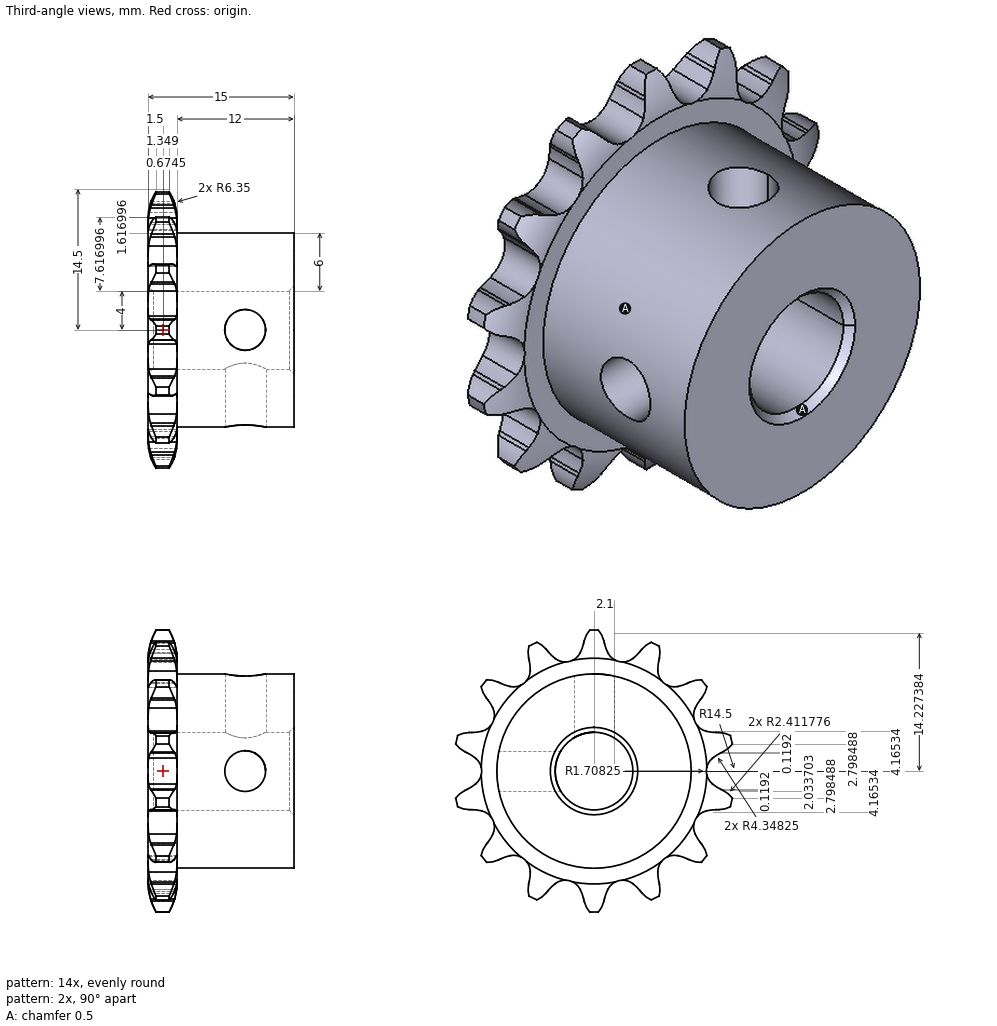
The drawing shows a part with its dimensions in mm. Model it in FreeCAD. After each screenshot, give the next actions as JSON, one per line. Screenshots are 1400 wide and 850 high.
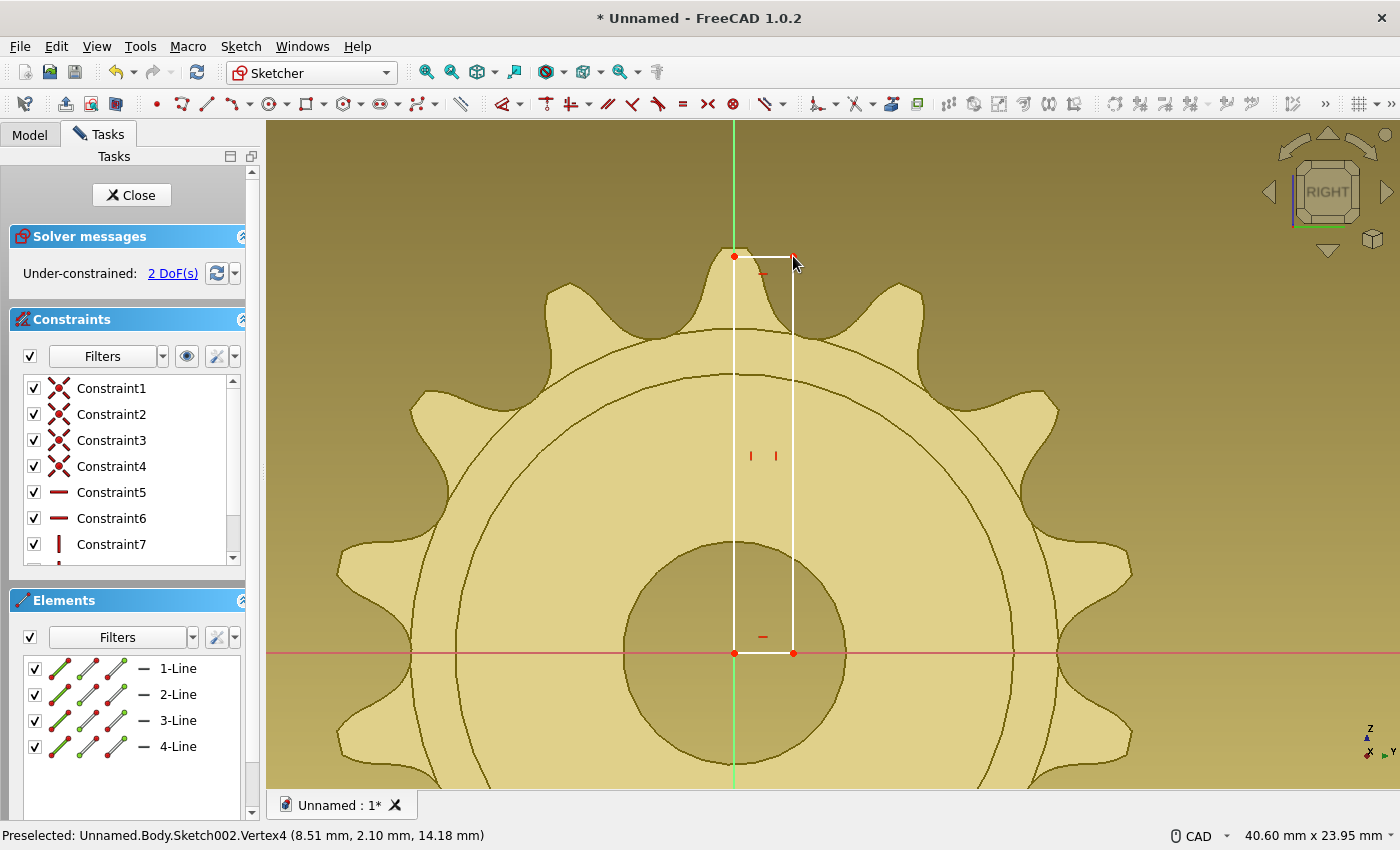
{"action": "left_click", "coordinate": [502, 104]}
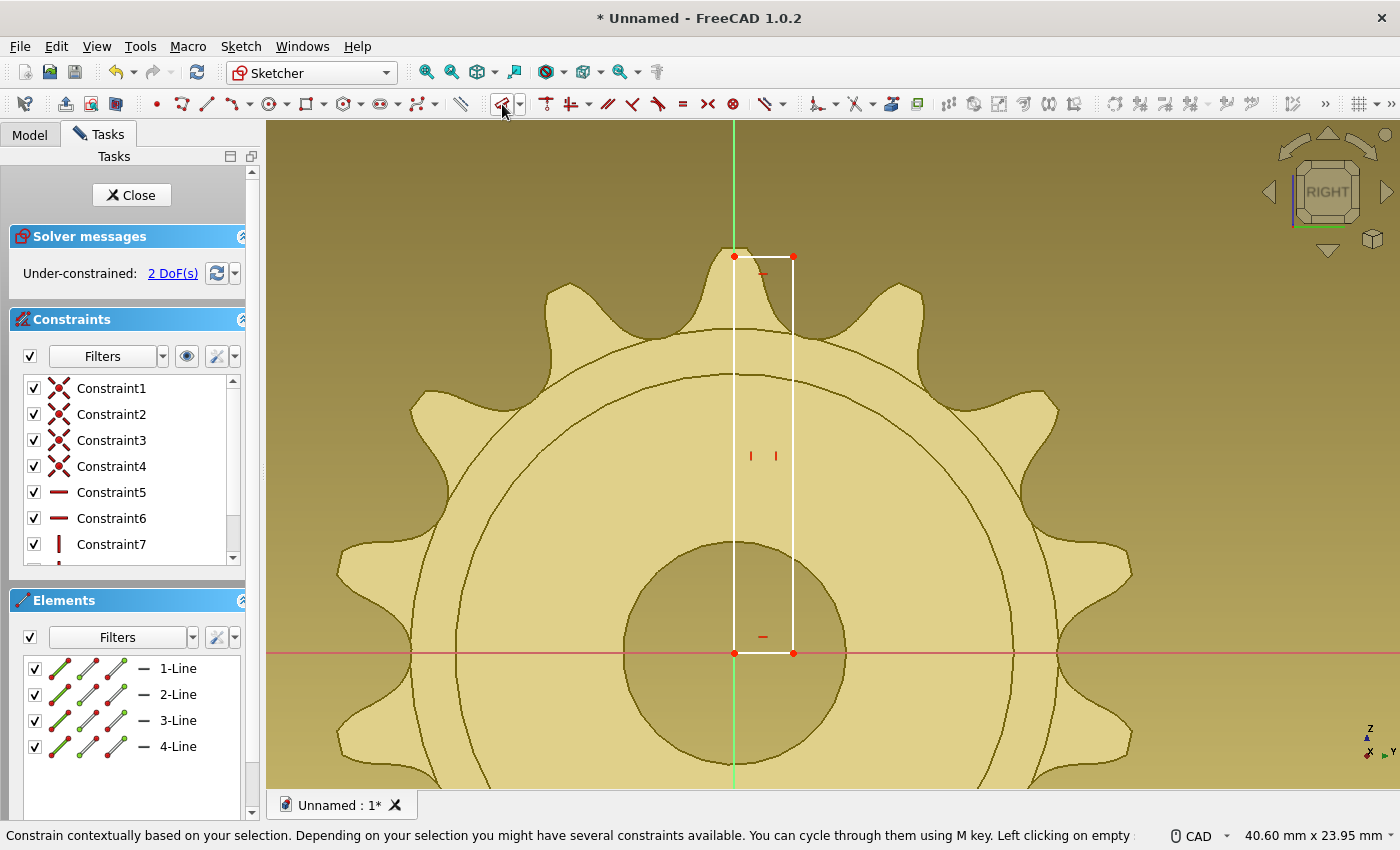
{"action": "left_click", "coordinate": [752, 653]}
{"action": "left_click", "coordinate": [764, 687]}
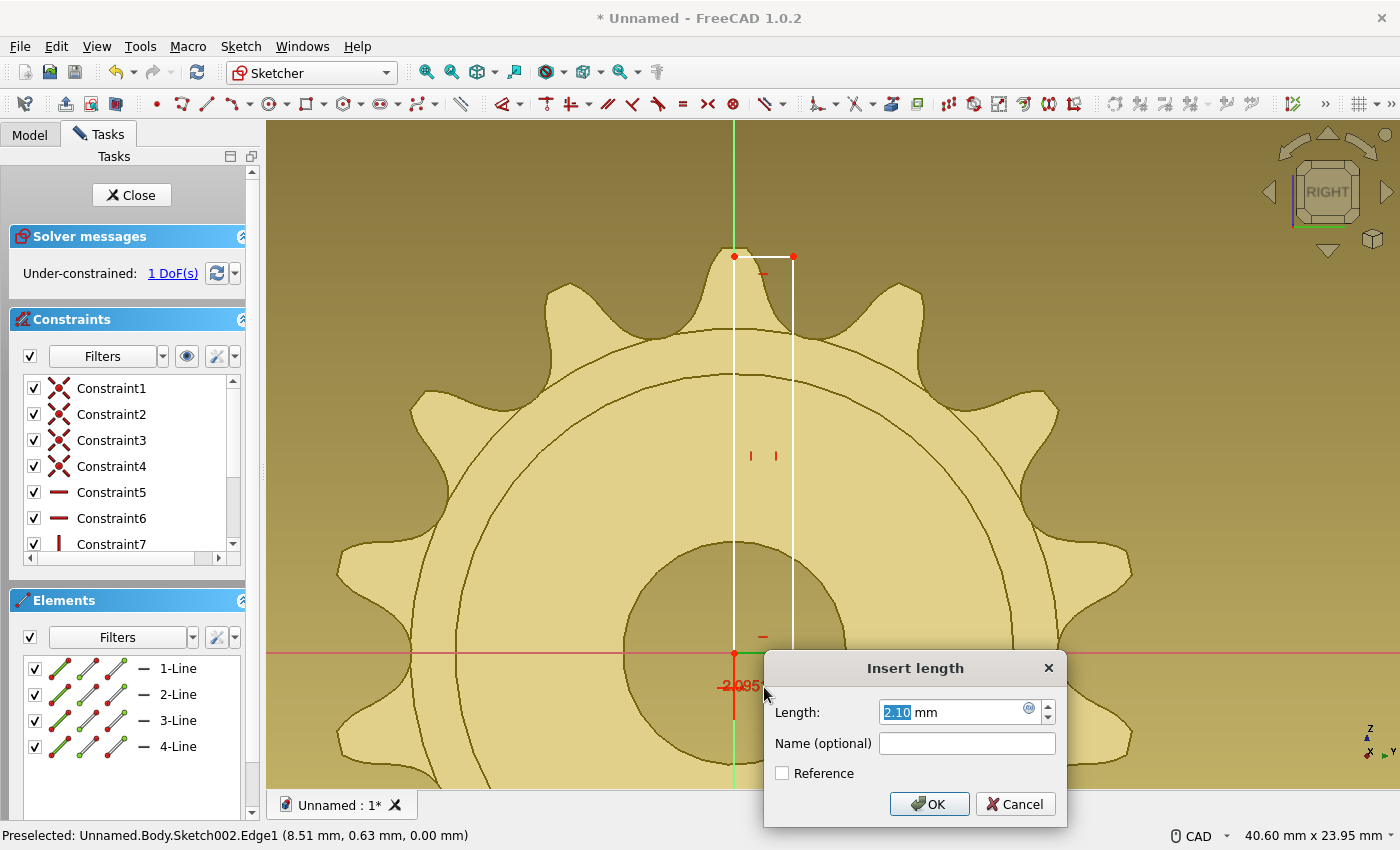
{"action": "type", "text": "2.1"}
{"action": "key", "text": "Return"}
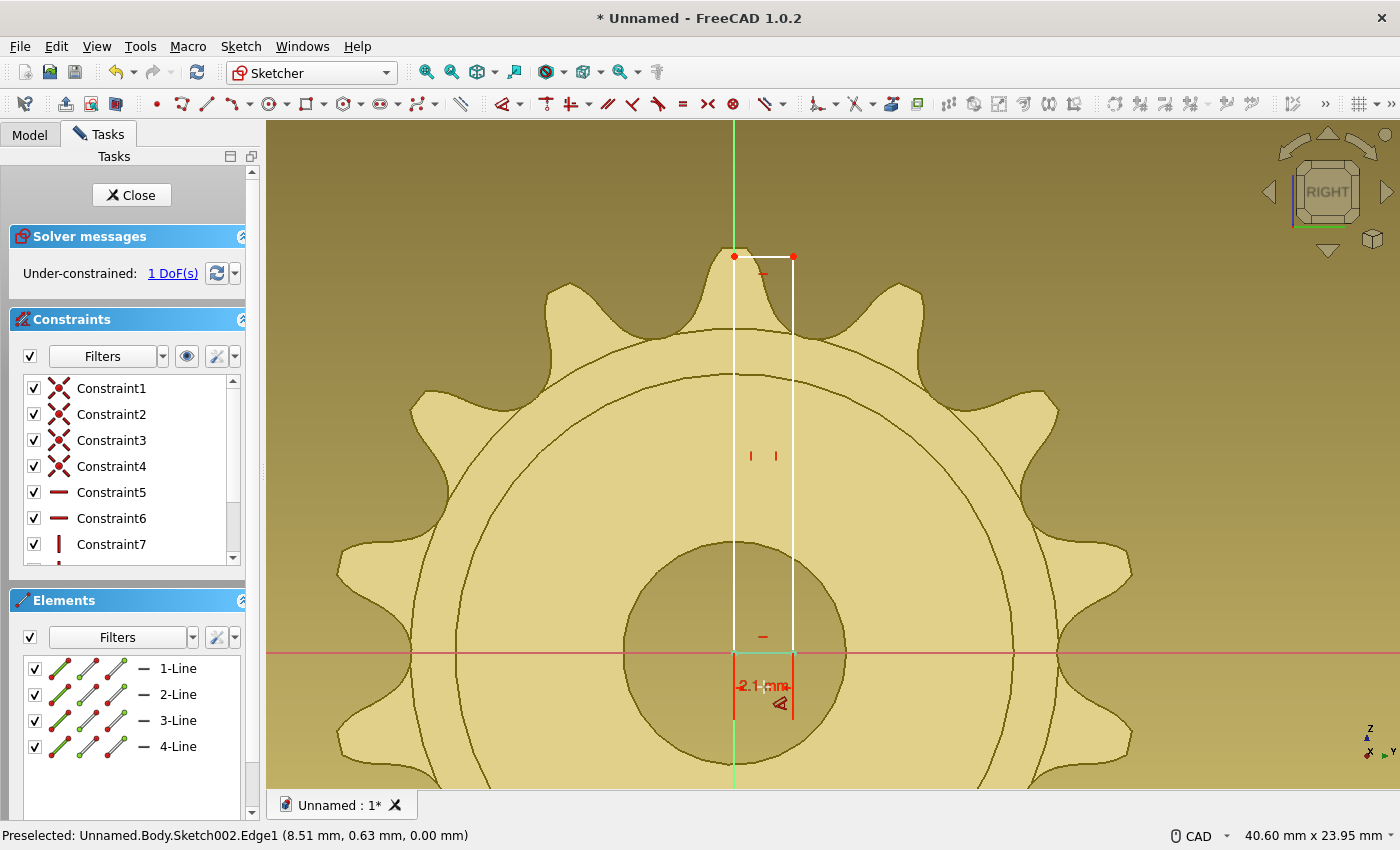
{"action": "left_click", "coordinate": [793, 534]}
{"action": "left_click", "coordinate": [827, 455]}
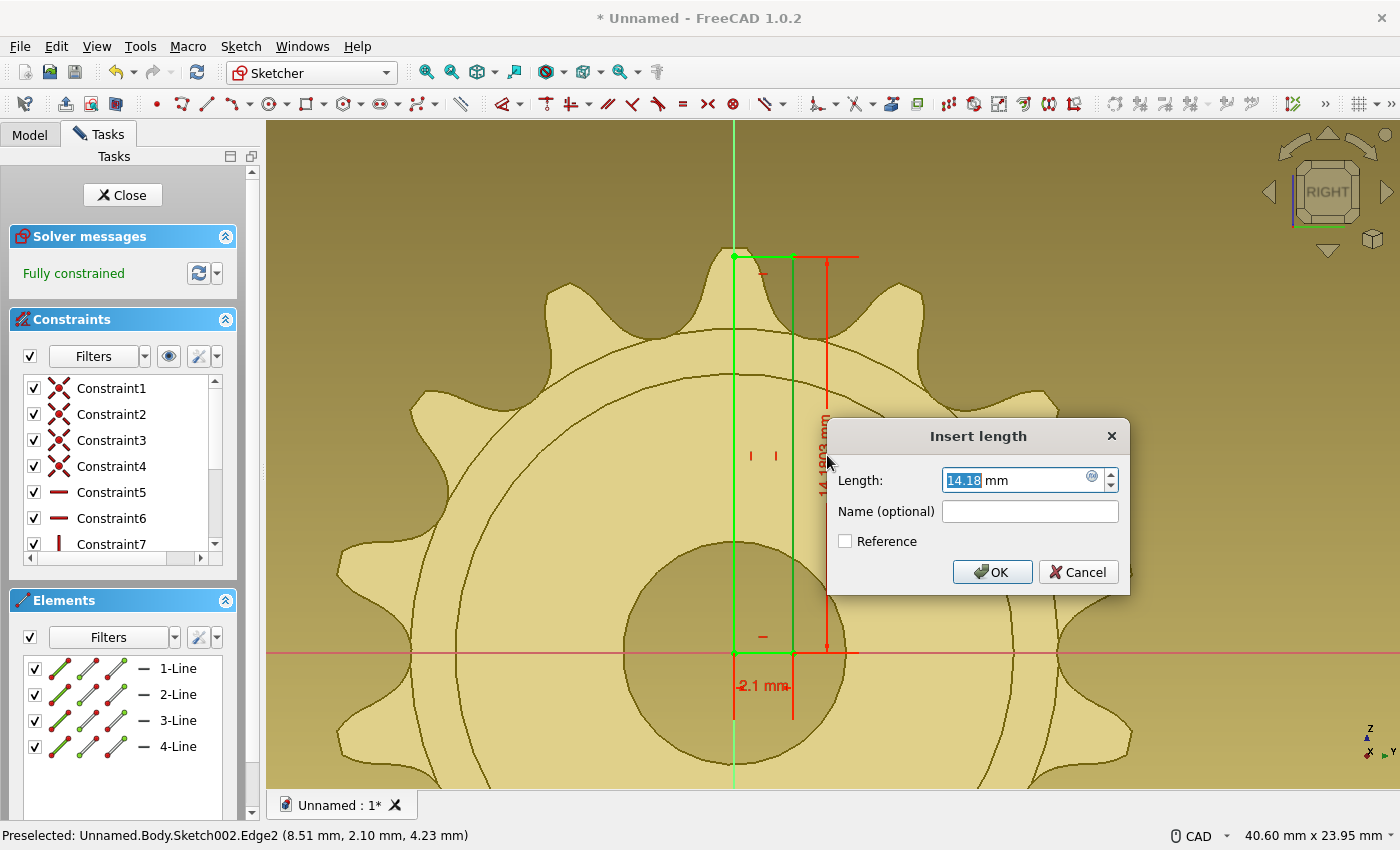
{"action": "type", "text": "14.227384"}
{"action": "key", "text": "Return"}
{"action": "key", "text": "Escape"}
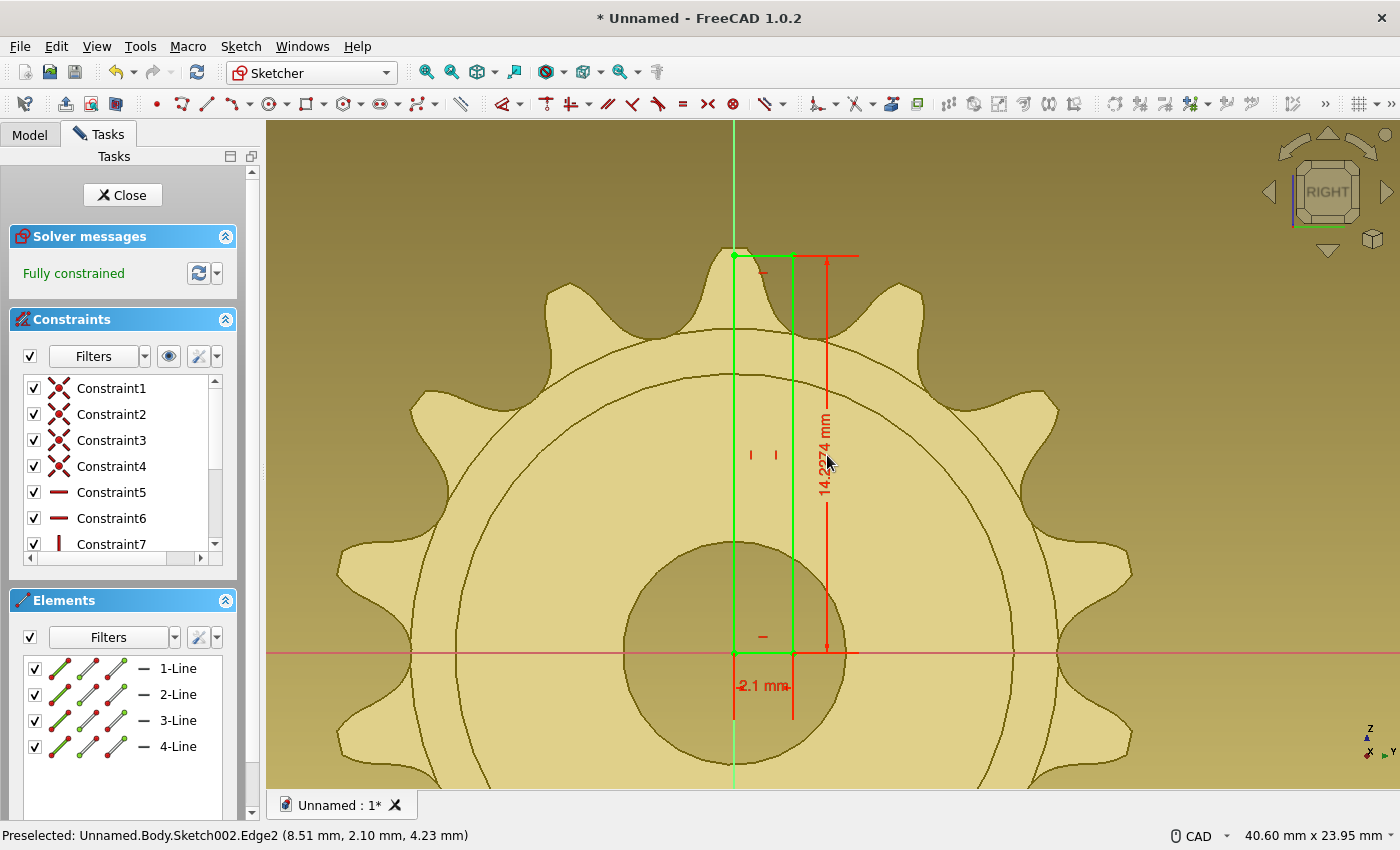
{"action": "left_click", "coordinate": [123, 195]}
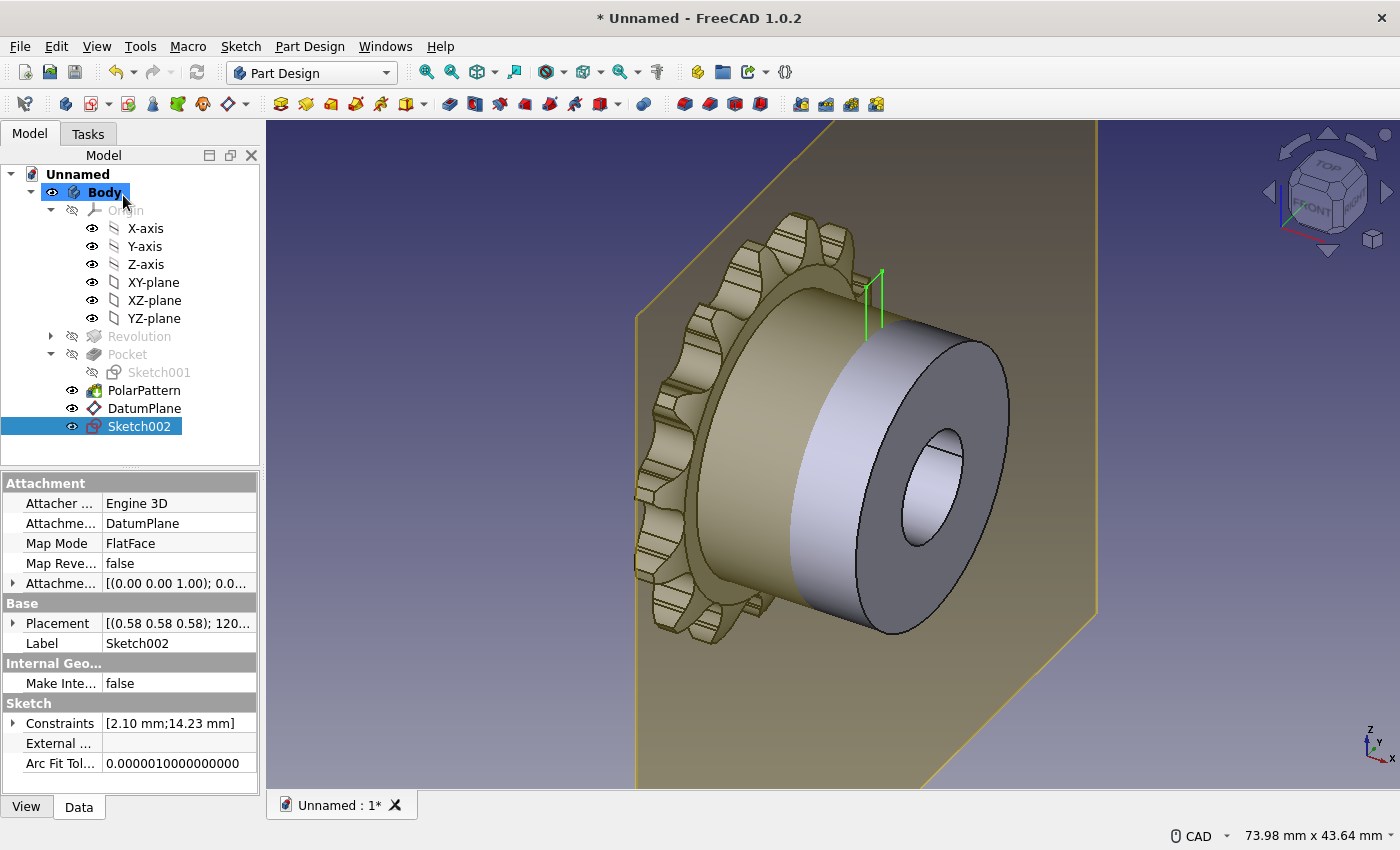
{"action": "left_click", "coordinate": [500, 104]}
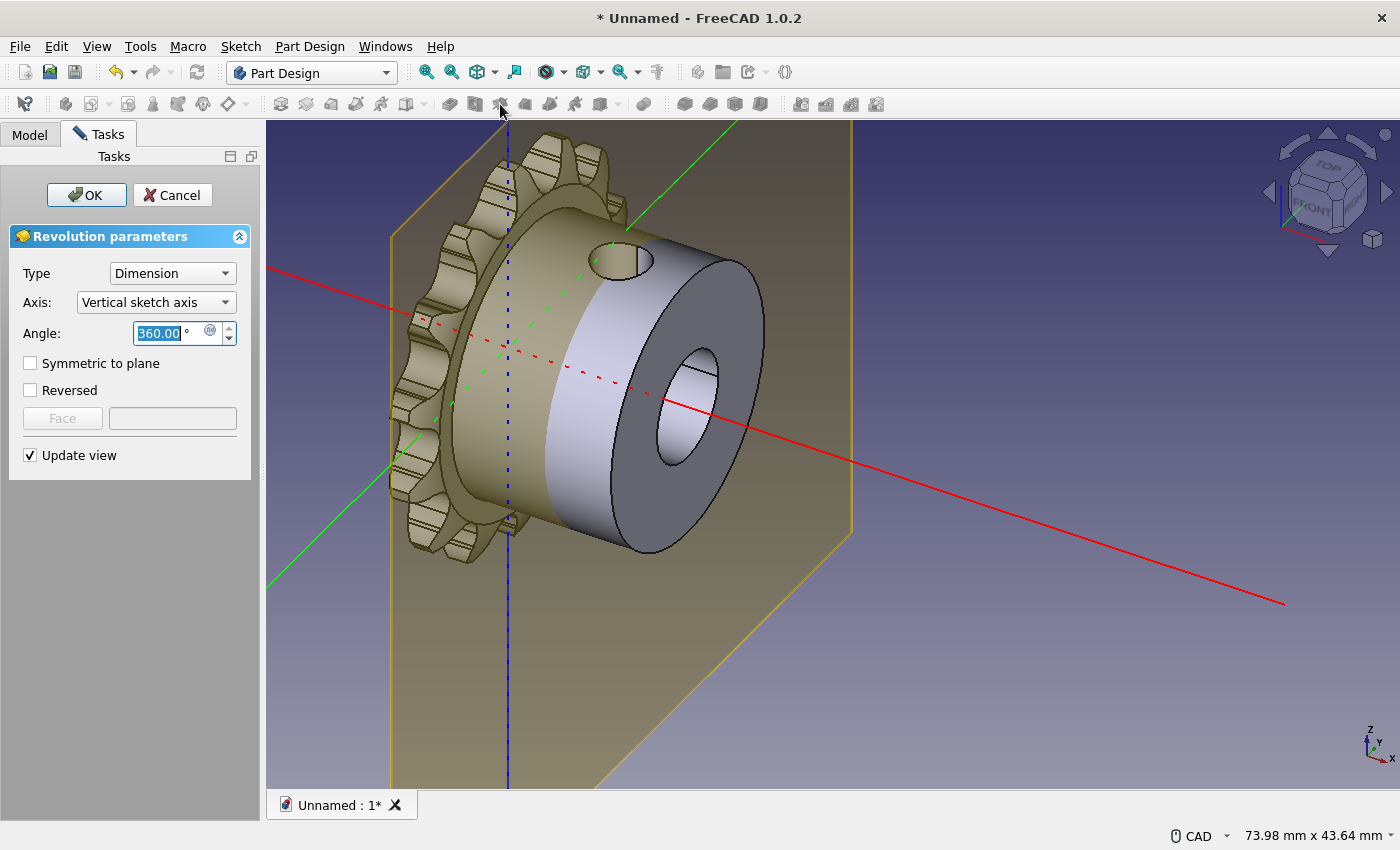
{"action": "left_click", "coordinate": [87, 195]}